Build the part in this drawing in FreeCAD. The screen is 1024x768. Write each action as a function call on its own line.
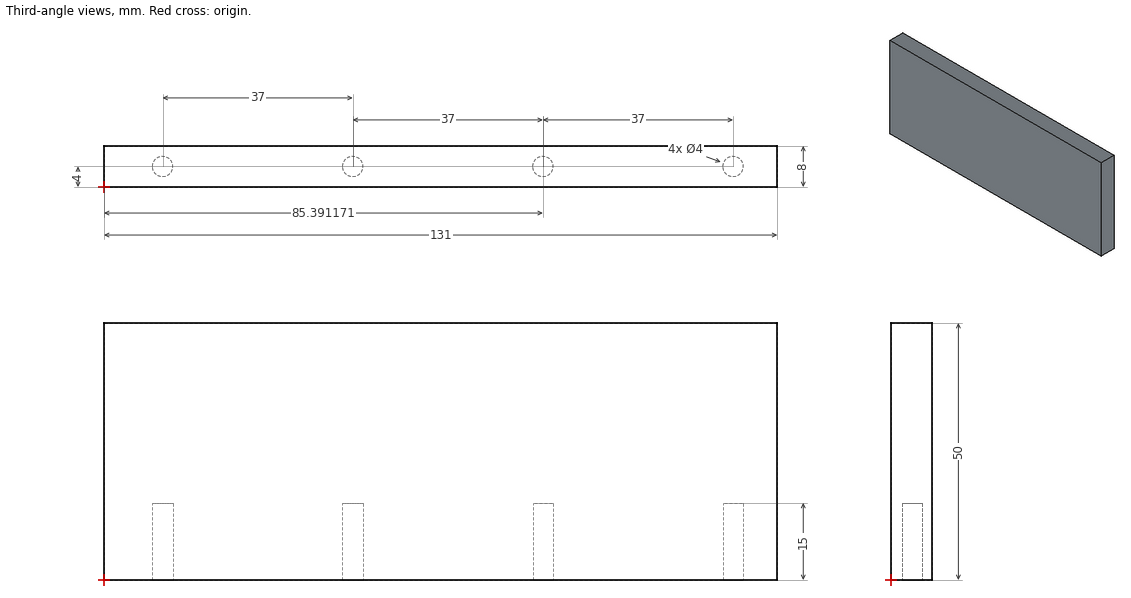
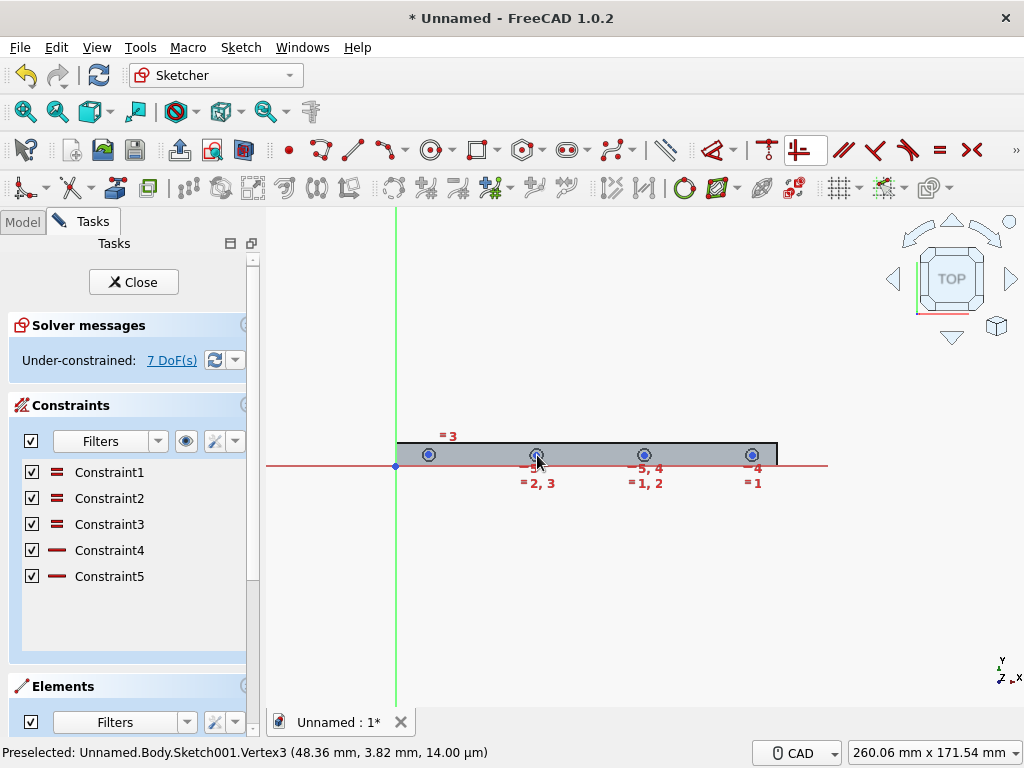
click(537, 455)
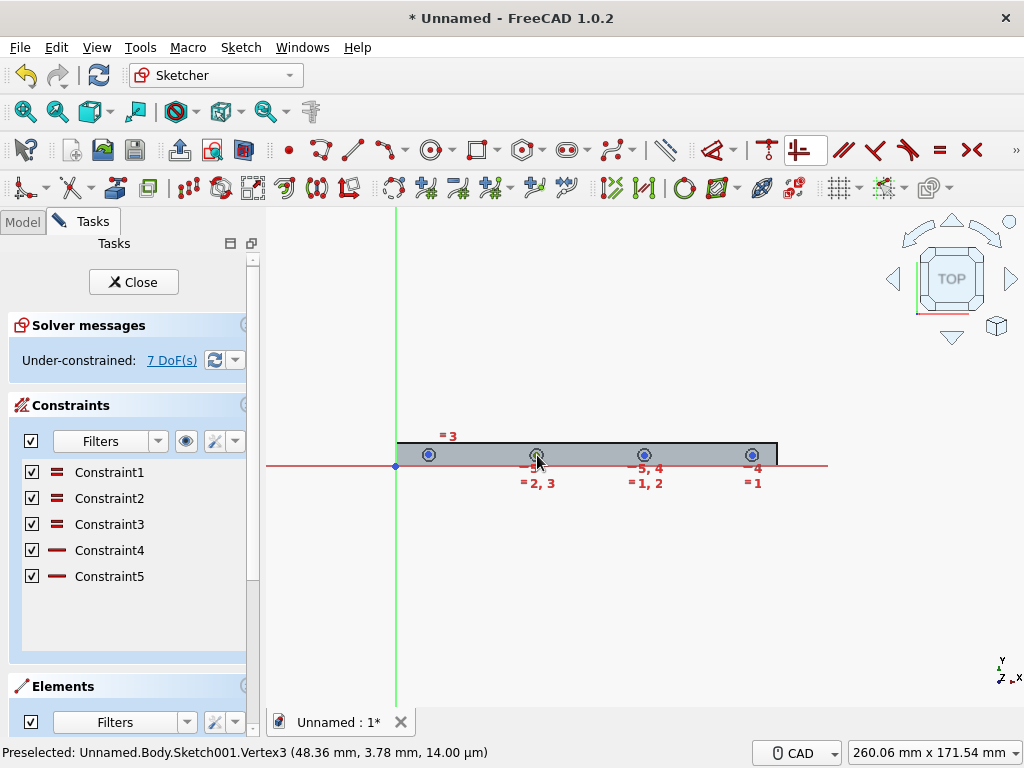
click(429, 455)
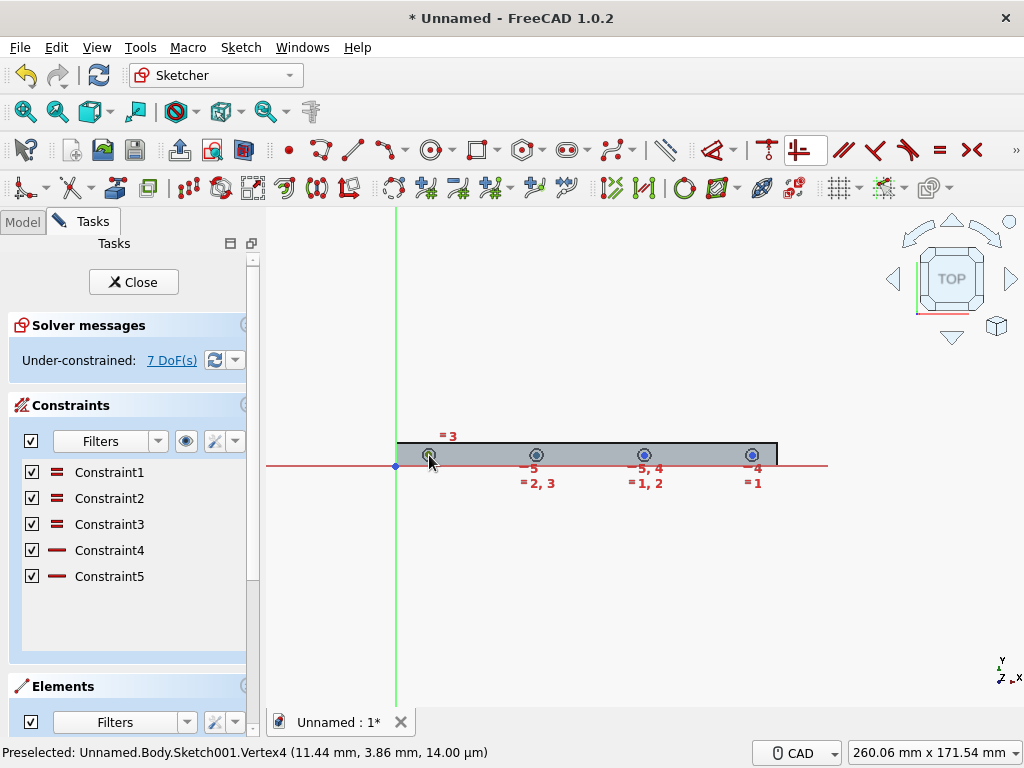
click(822, 150)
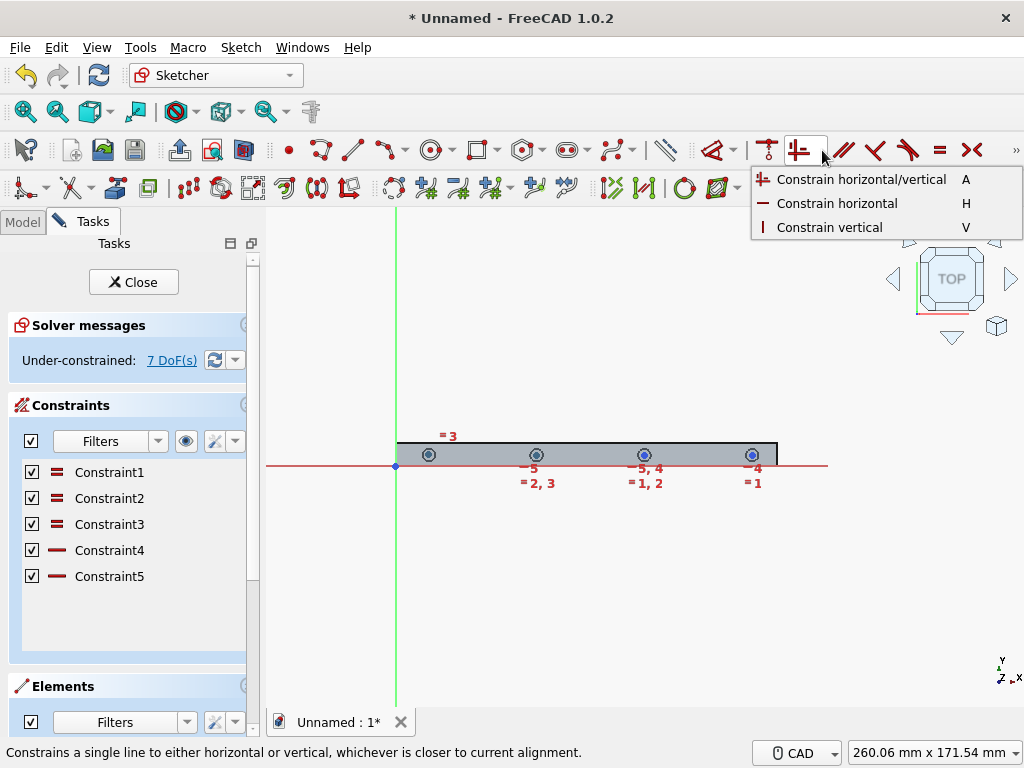
click(887, 203)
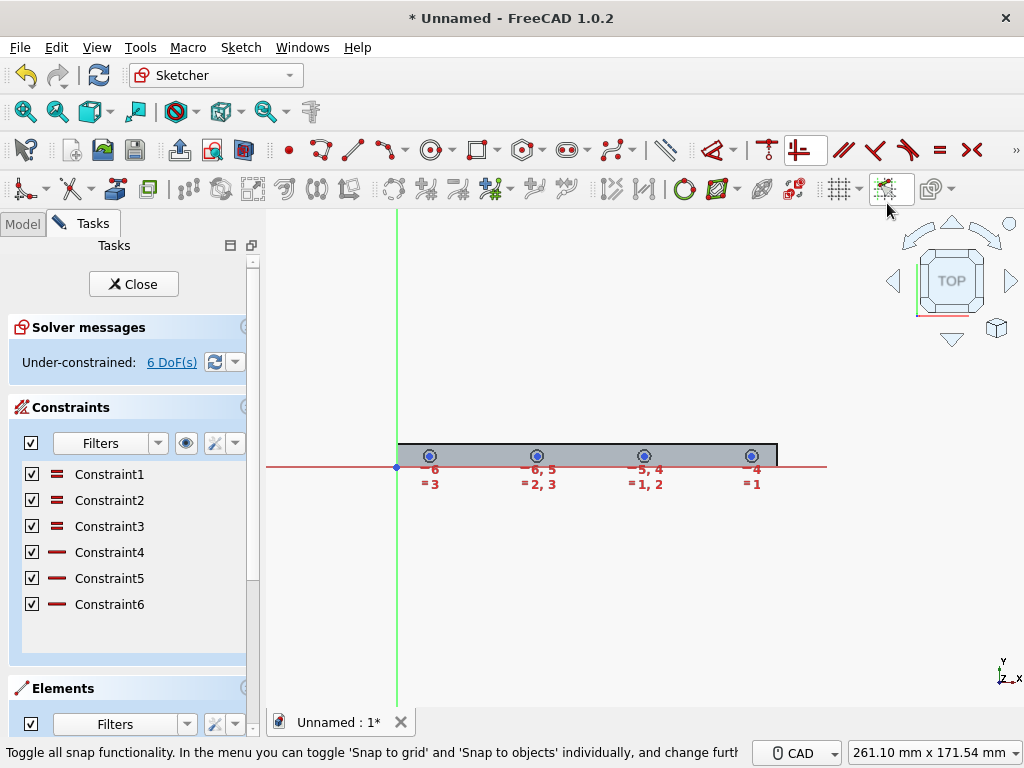
click(712, 150)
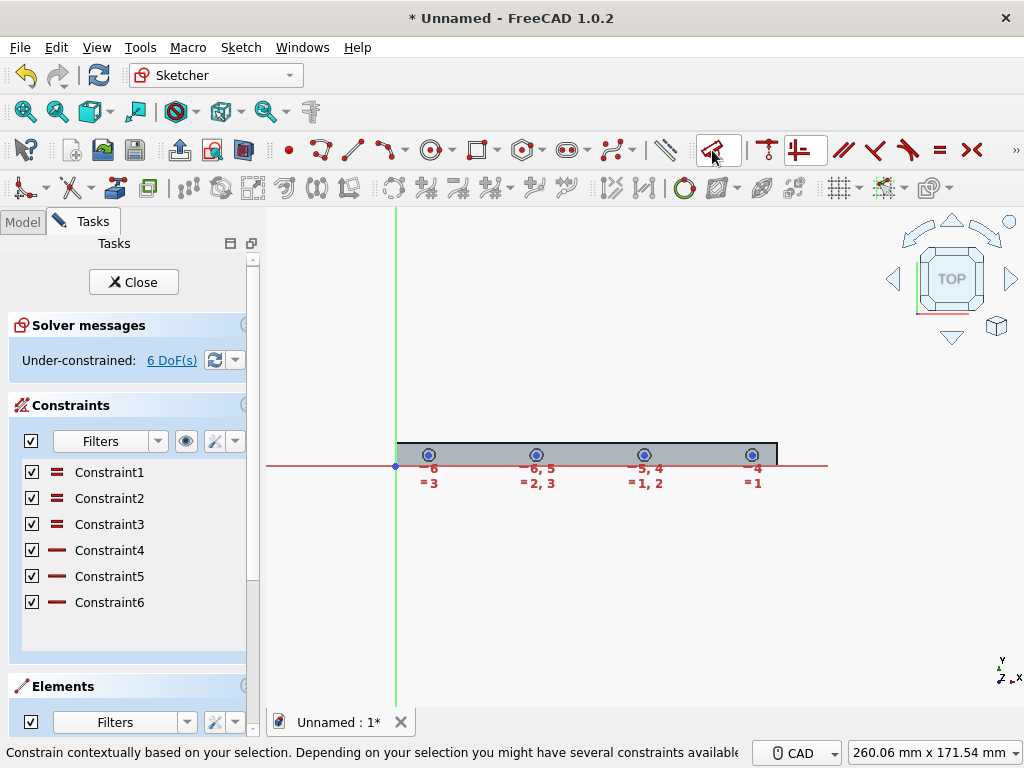
scroll(748, 451, up, 7)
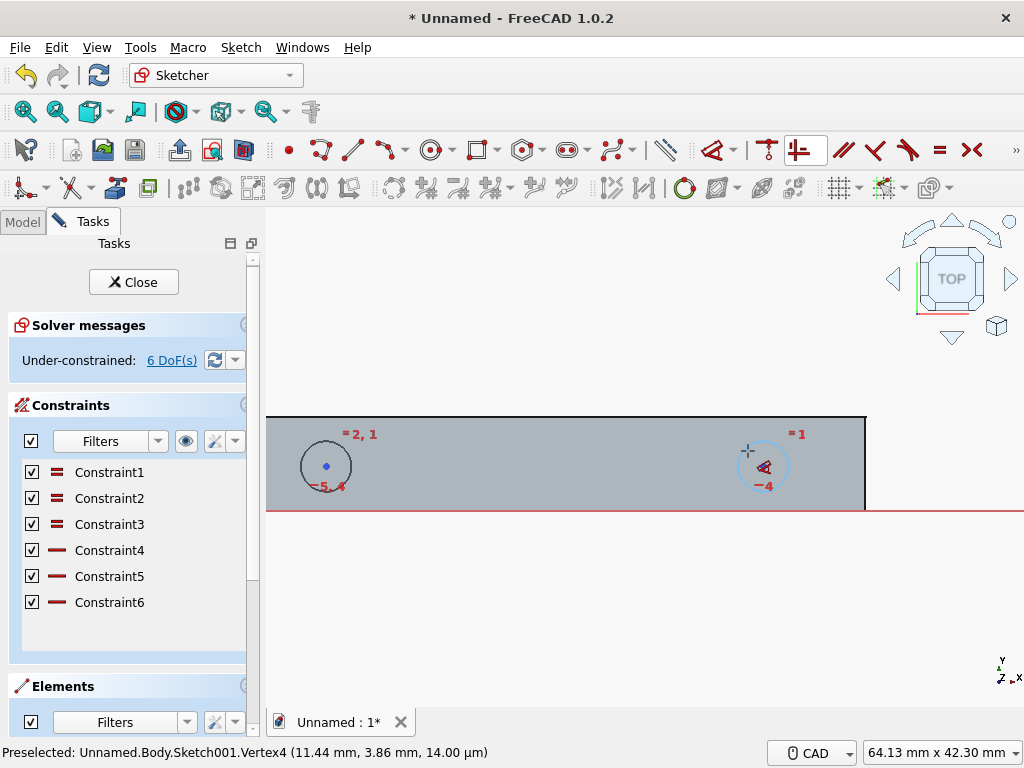
click(745, 449)
click(722, 427)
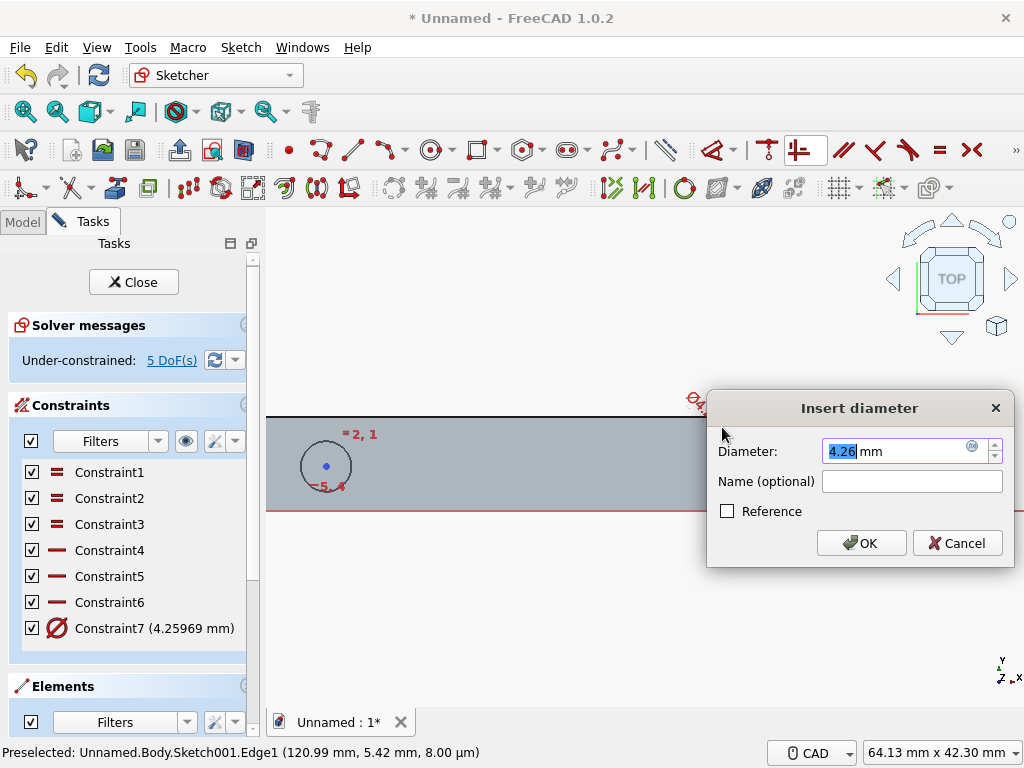
text(4)
key(Return)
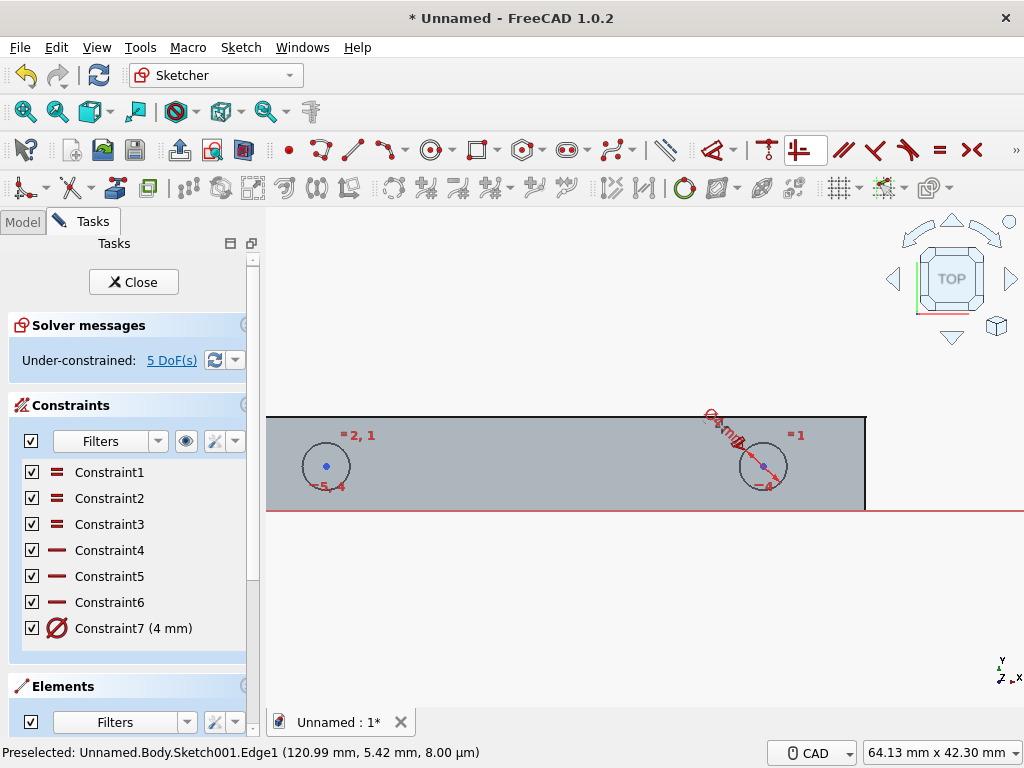
click(763, 466)
click(797, 489)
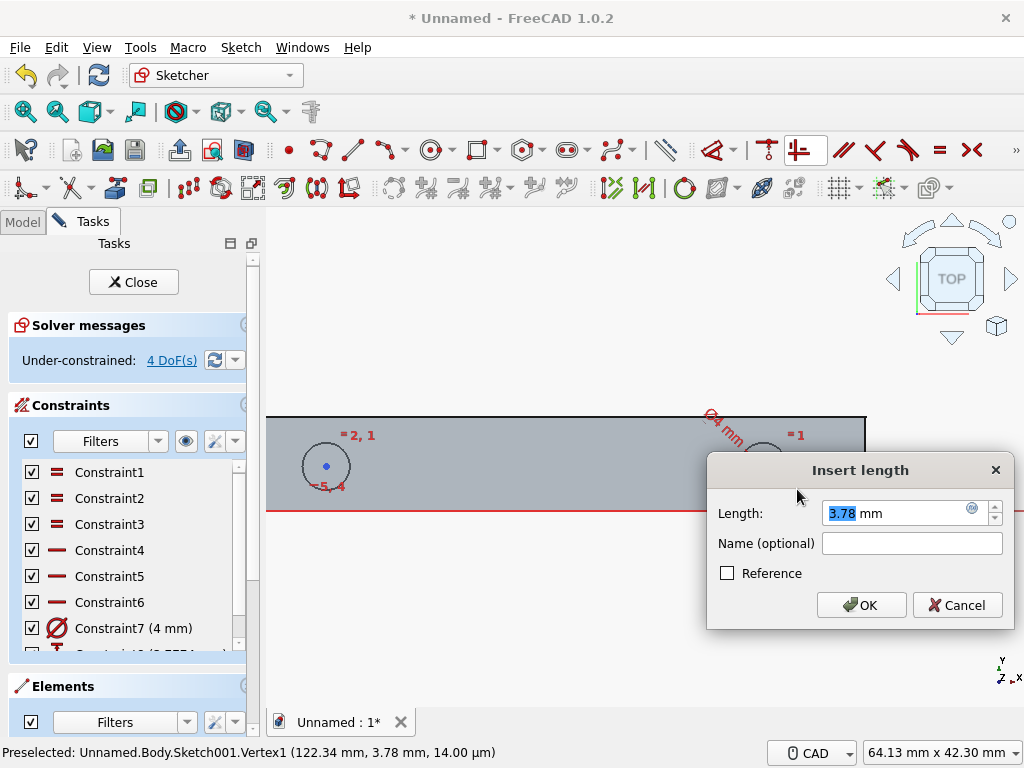
text(4)
key(Return)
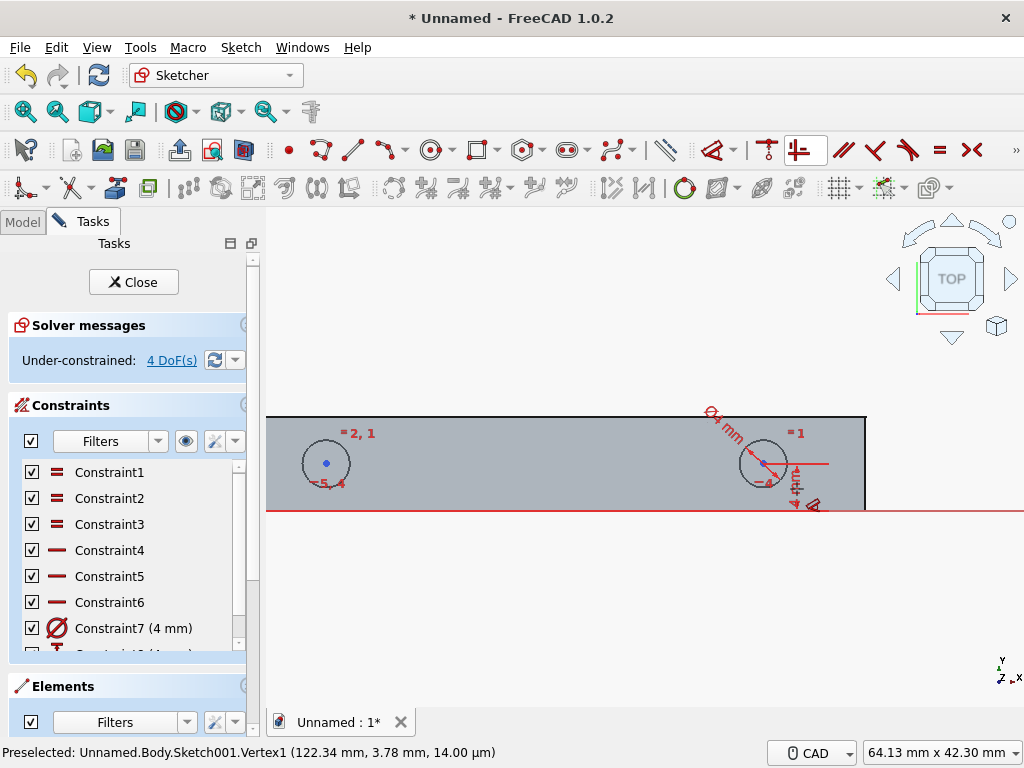
scroll(748, 451, down, 7)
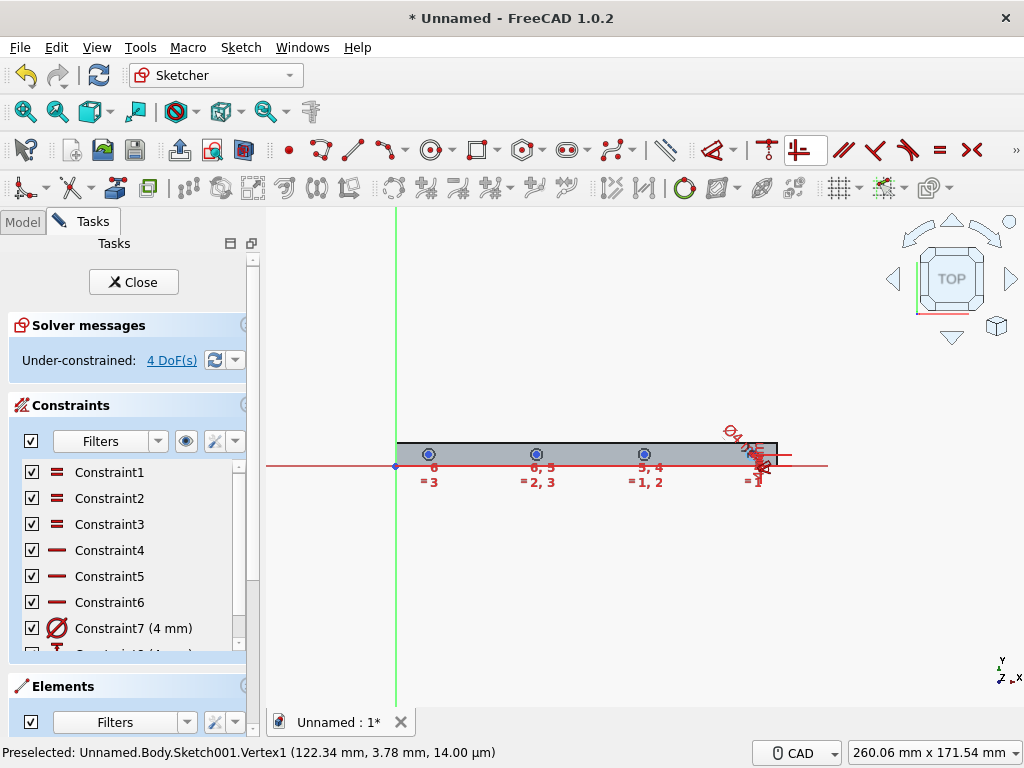
click(752, 455)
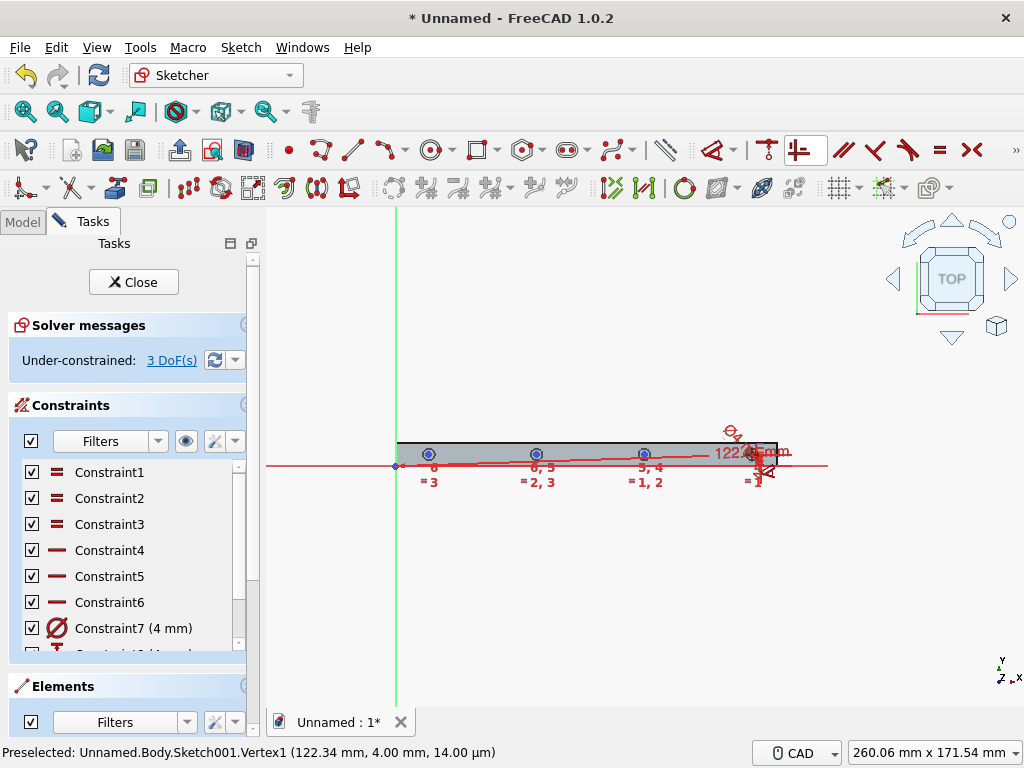
click(644, 455)
click(698, 421)